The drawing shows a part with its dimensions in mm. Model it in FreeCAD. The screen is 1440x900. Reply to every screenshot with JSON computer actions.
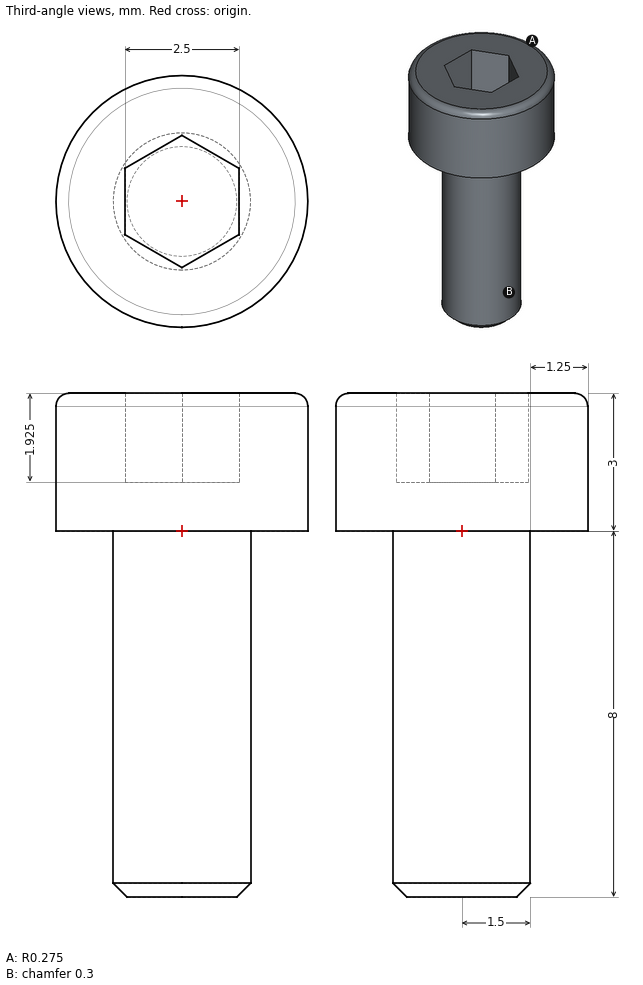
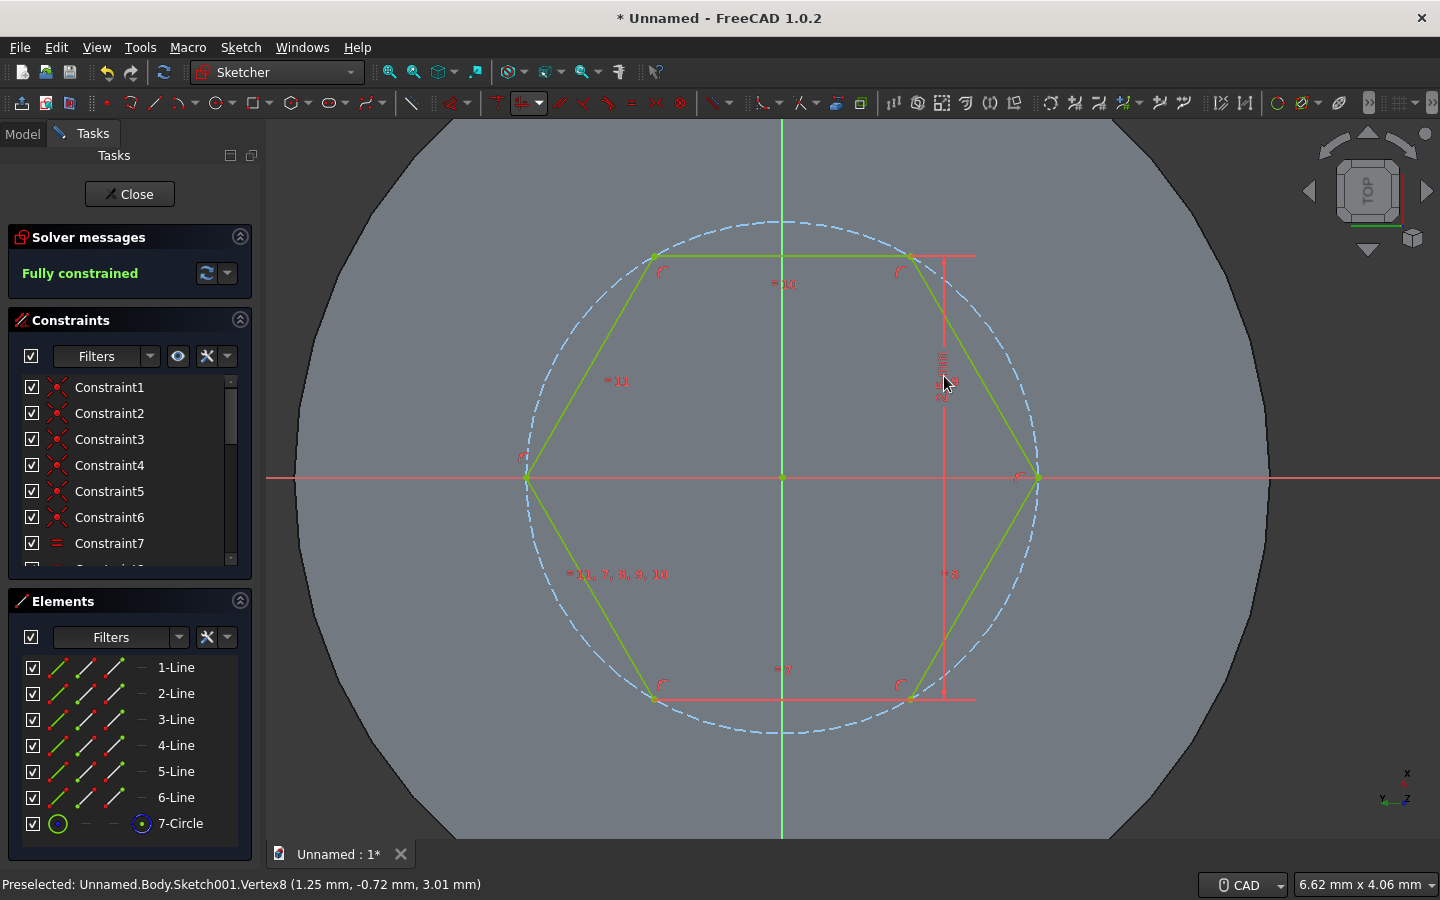
{"action": "left_click", "coordinate": [130, 194]}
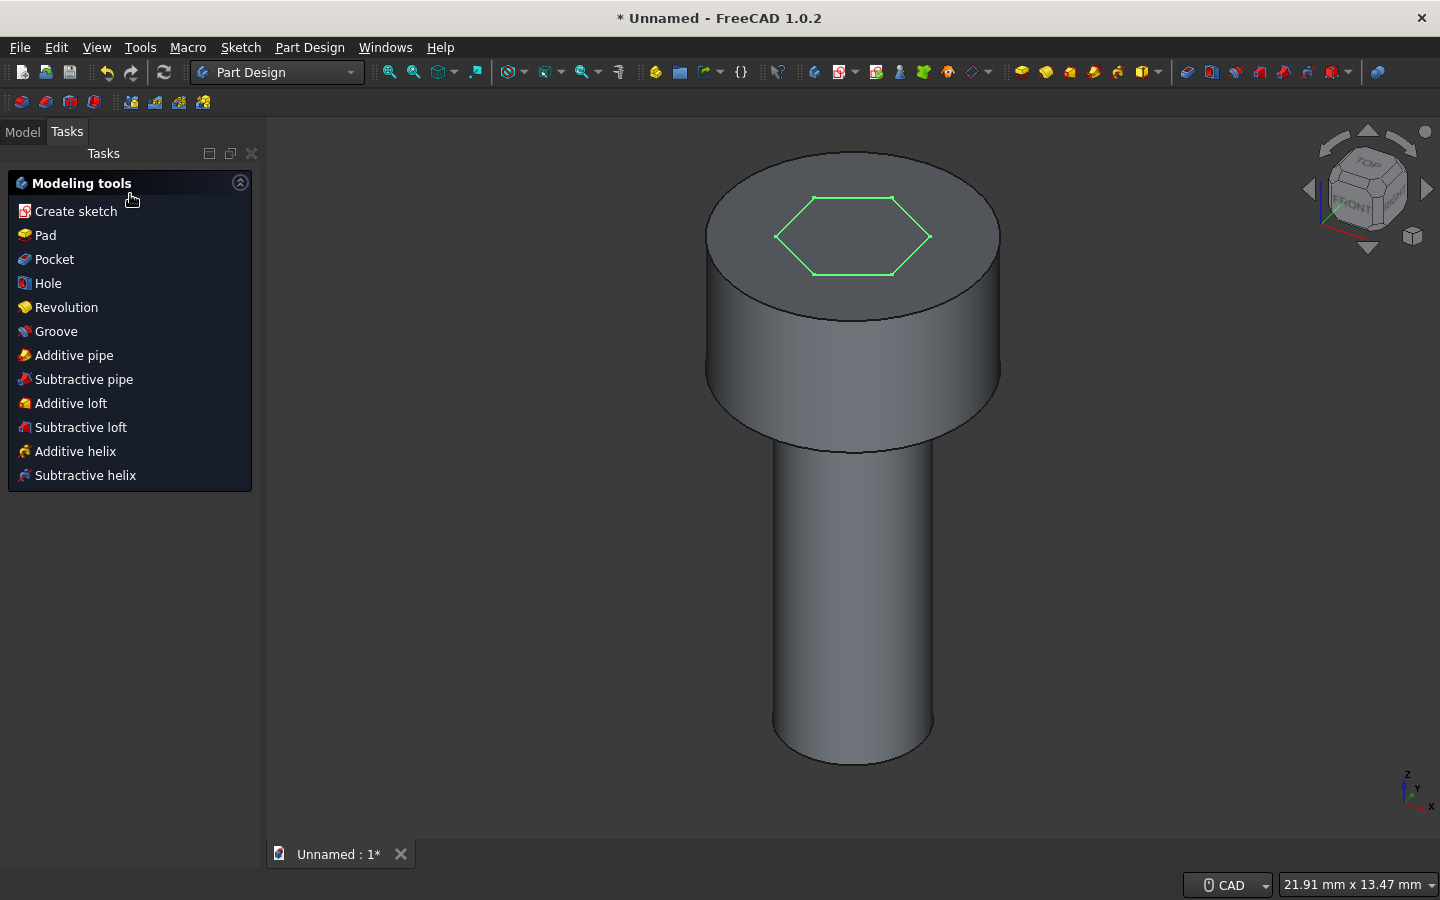
{"action": "left_click", "coordinate": [1188, 72]}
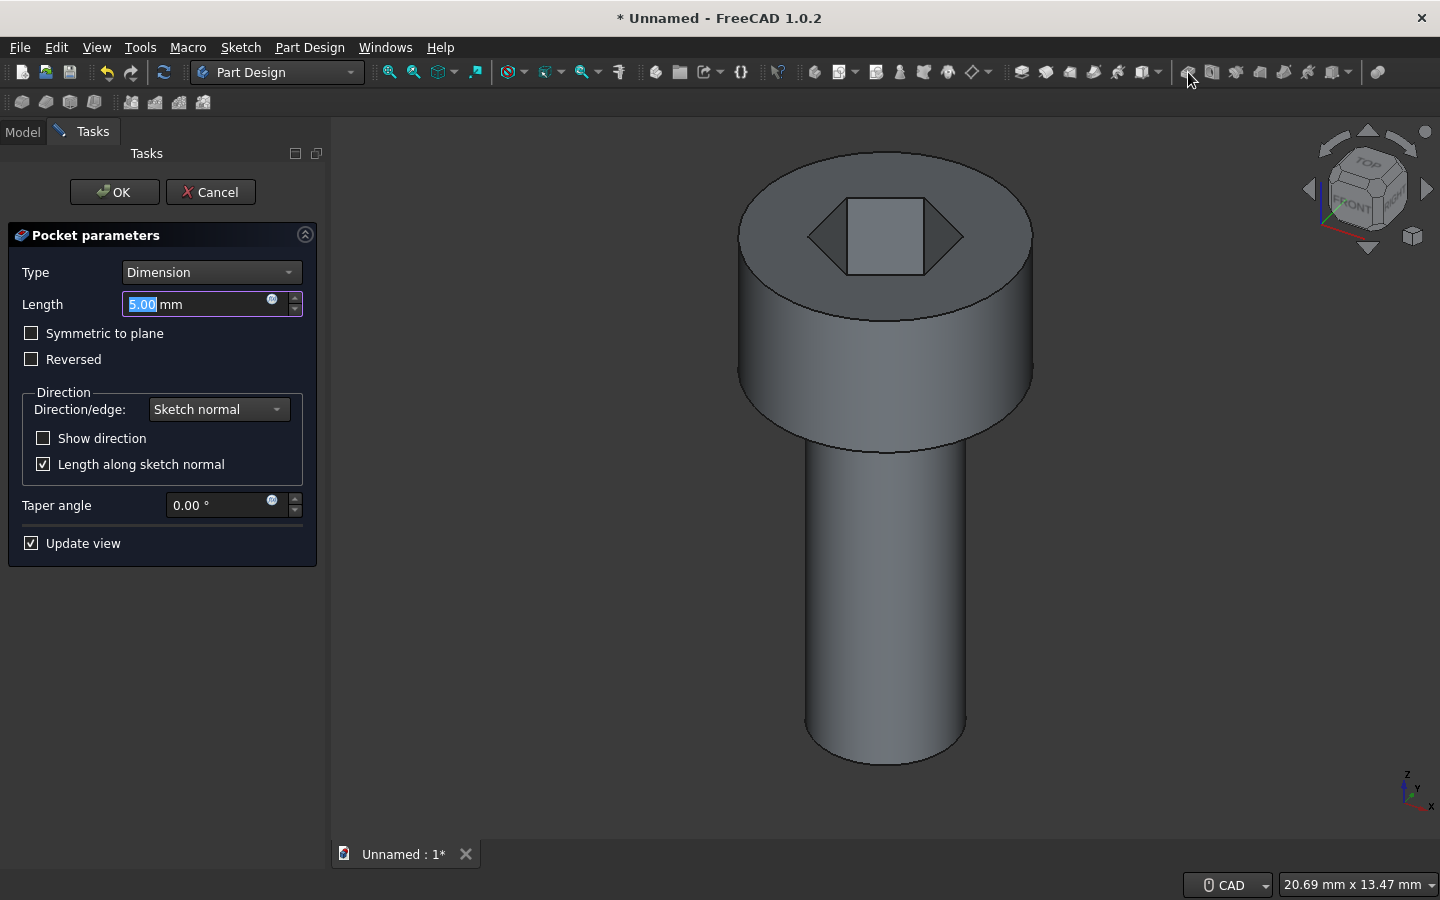
{"action": "type", "text": "1.925"}
{"action": "key", "text": "Tab"}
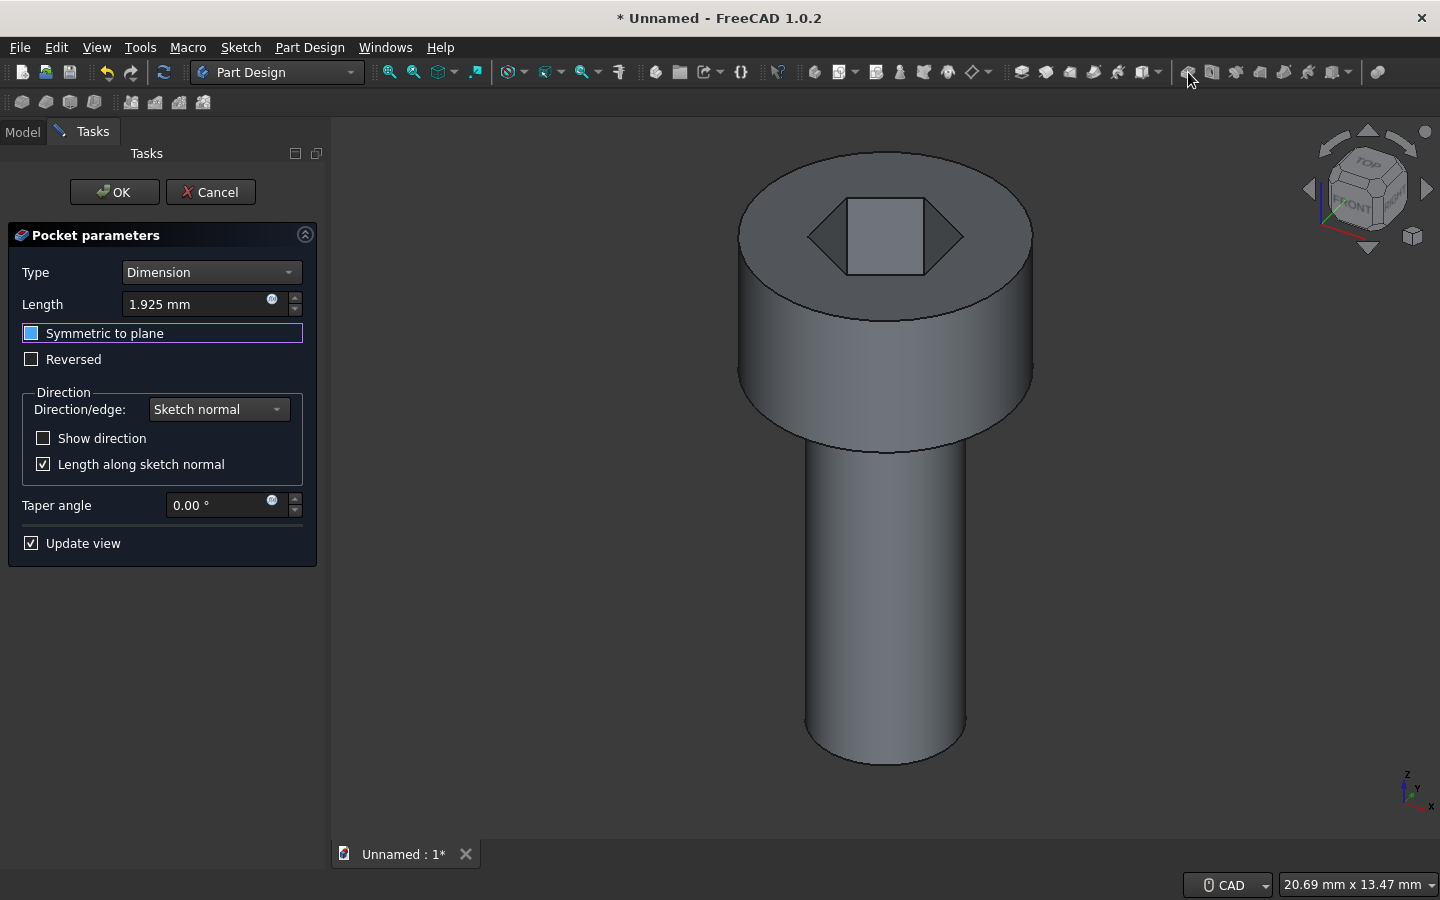
{"action": "left_click", "coordinate": [115, 192]}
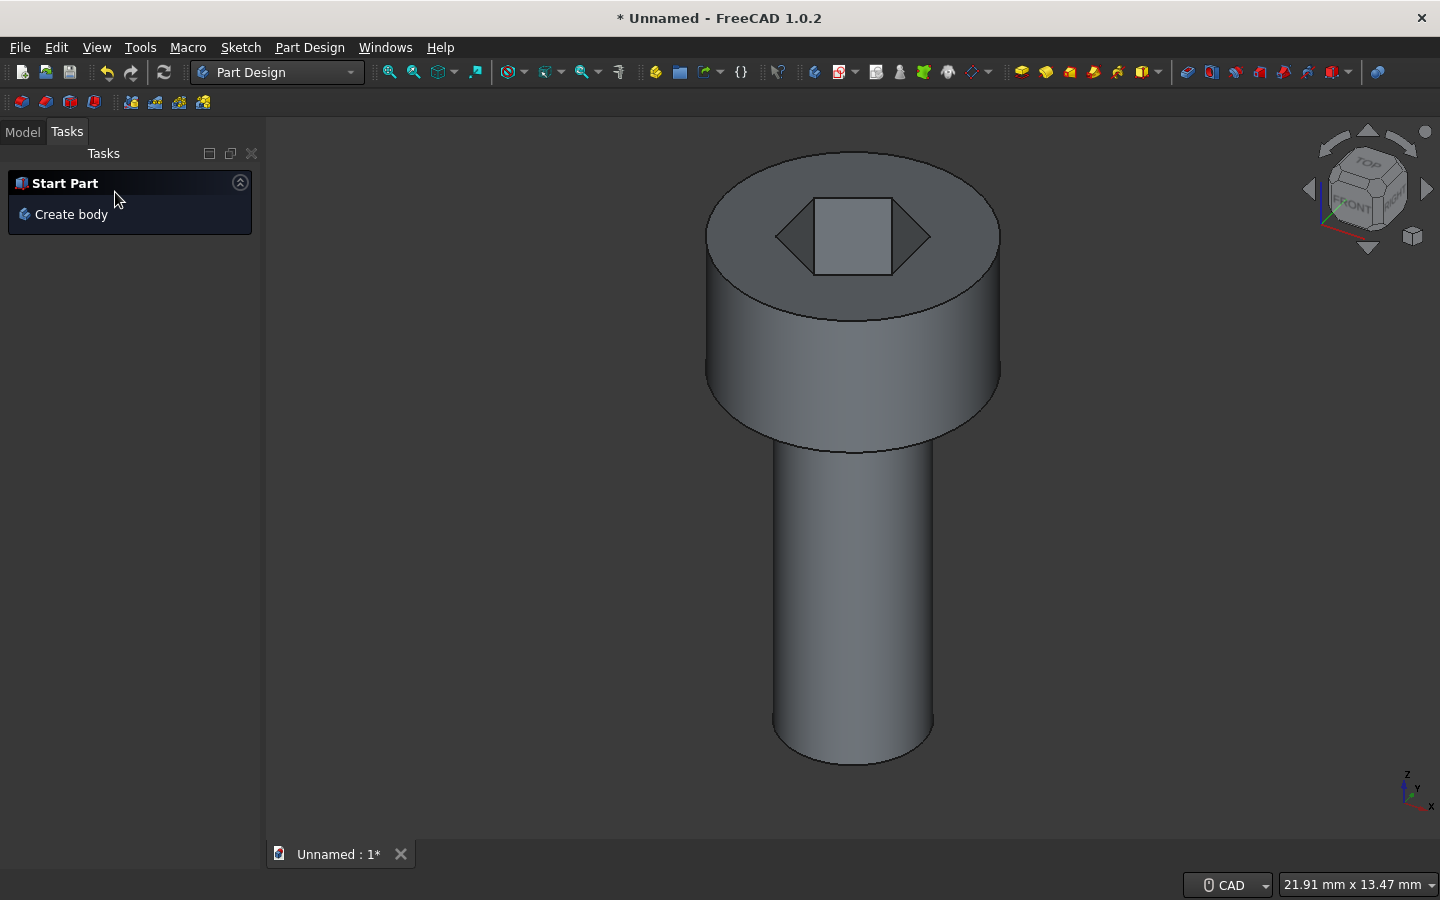
{"action": "left_click", "coordinate": [779, 309]}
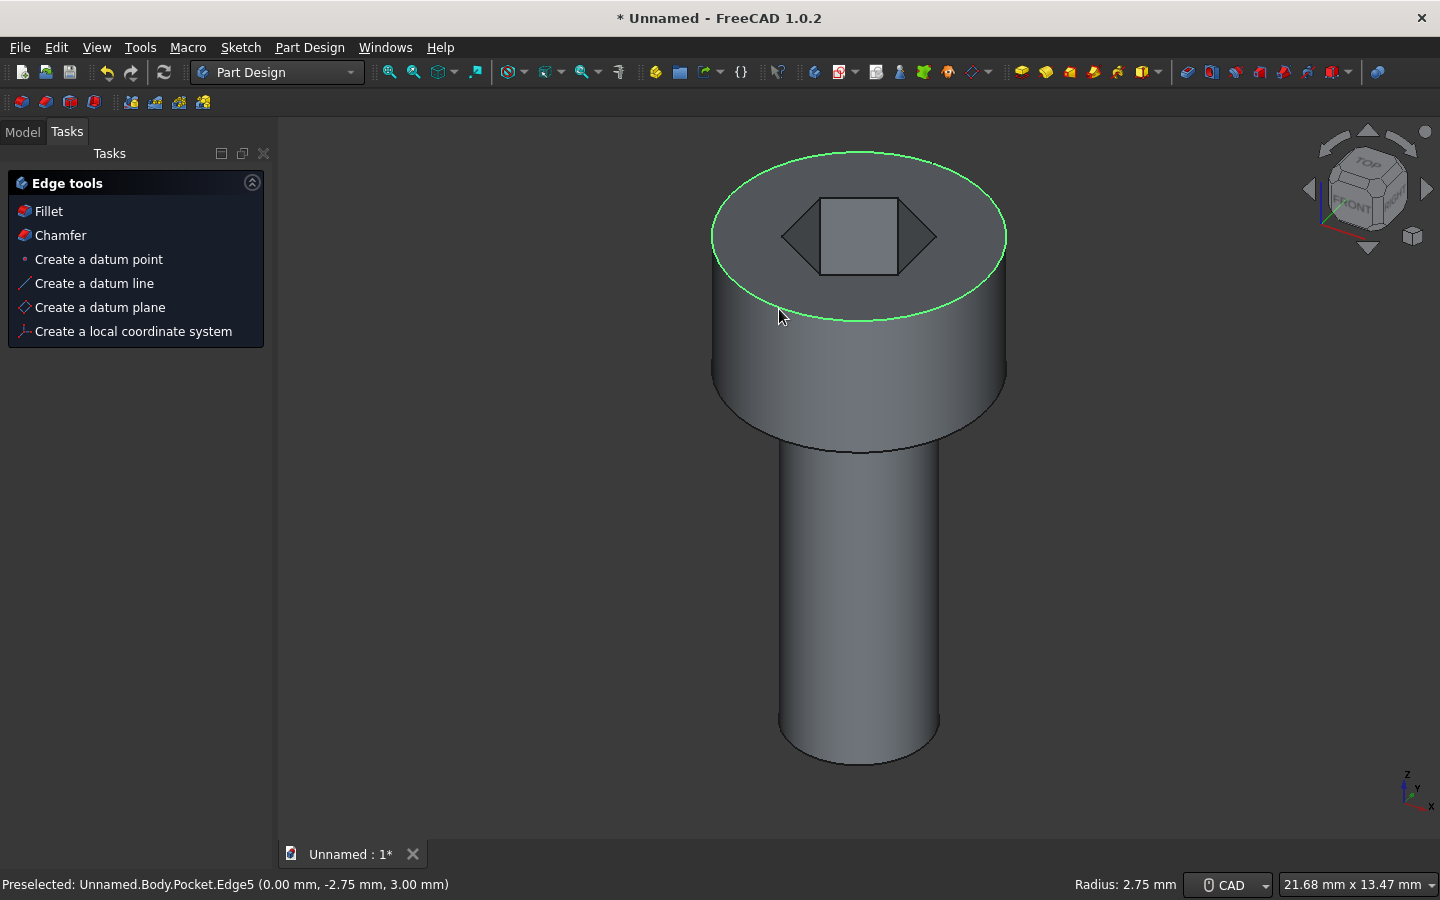
{"action": "left_click", "coordinate": [22, 102]}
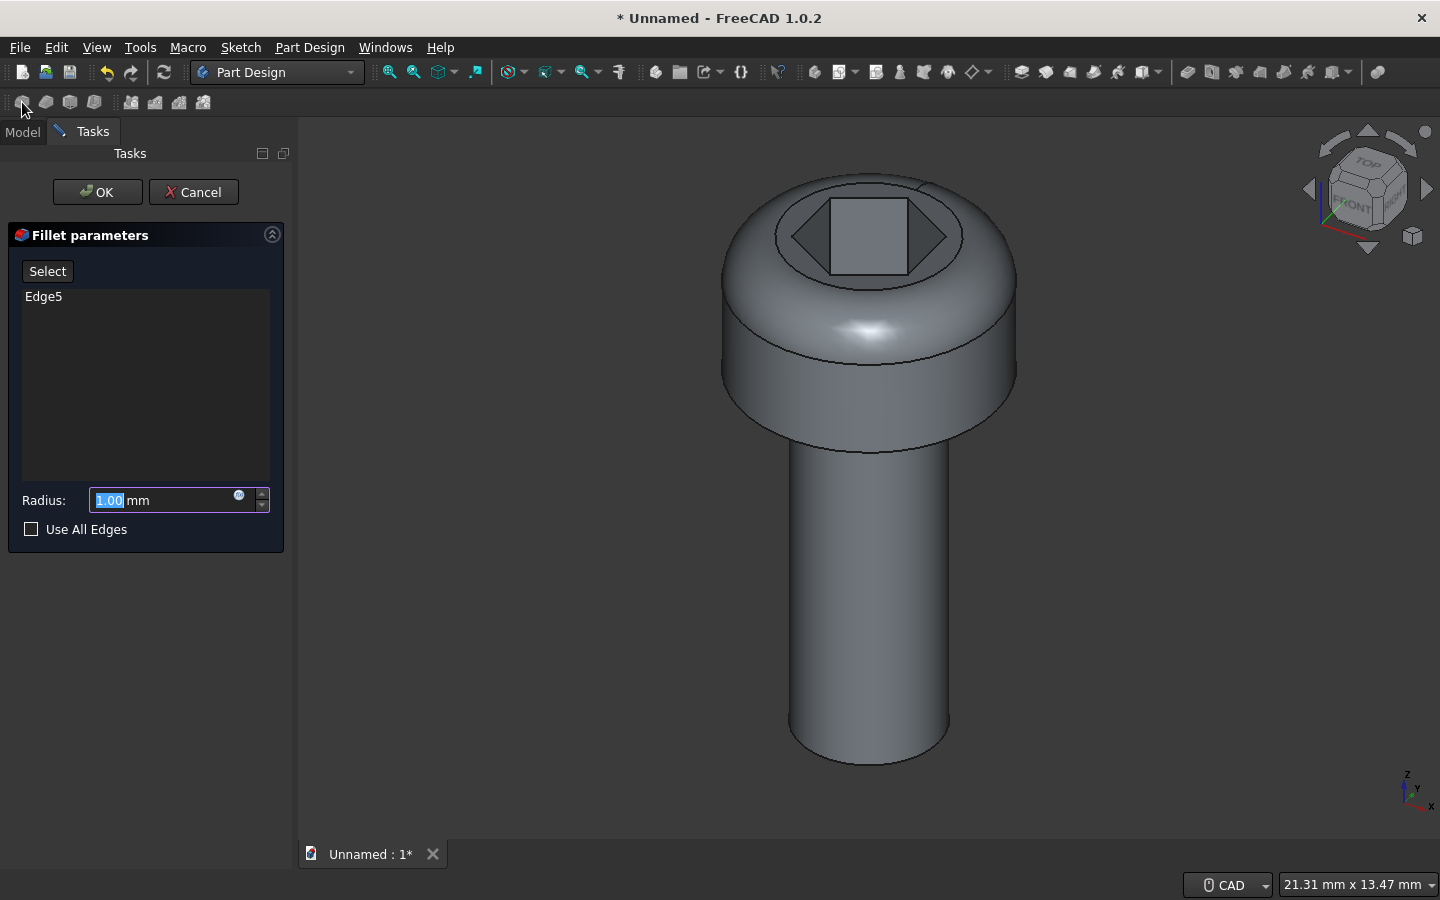
{"action": "type", "text": "0.275"}
{"action": "key", "text": "Tab"}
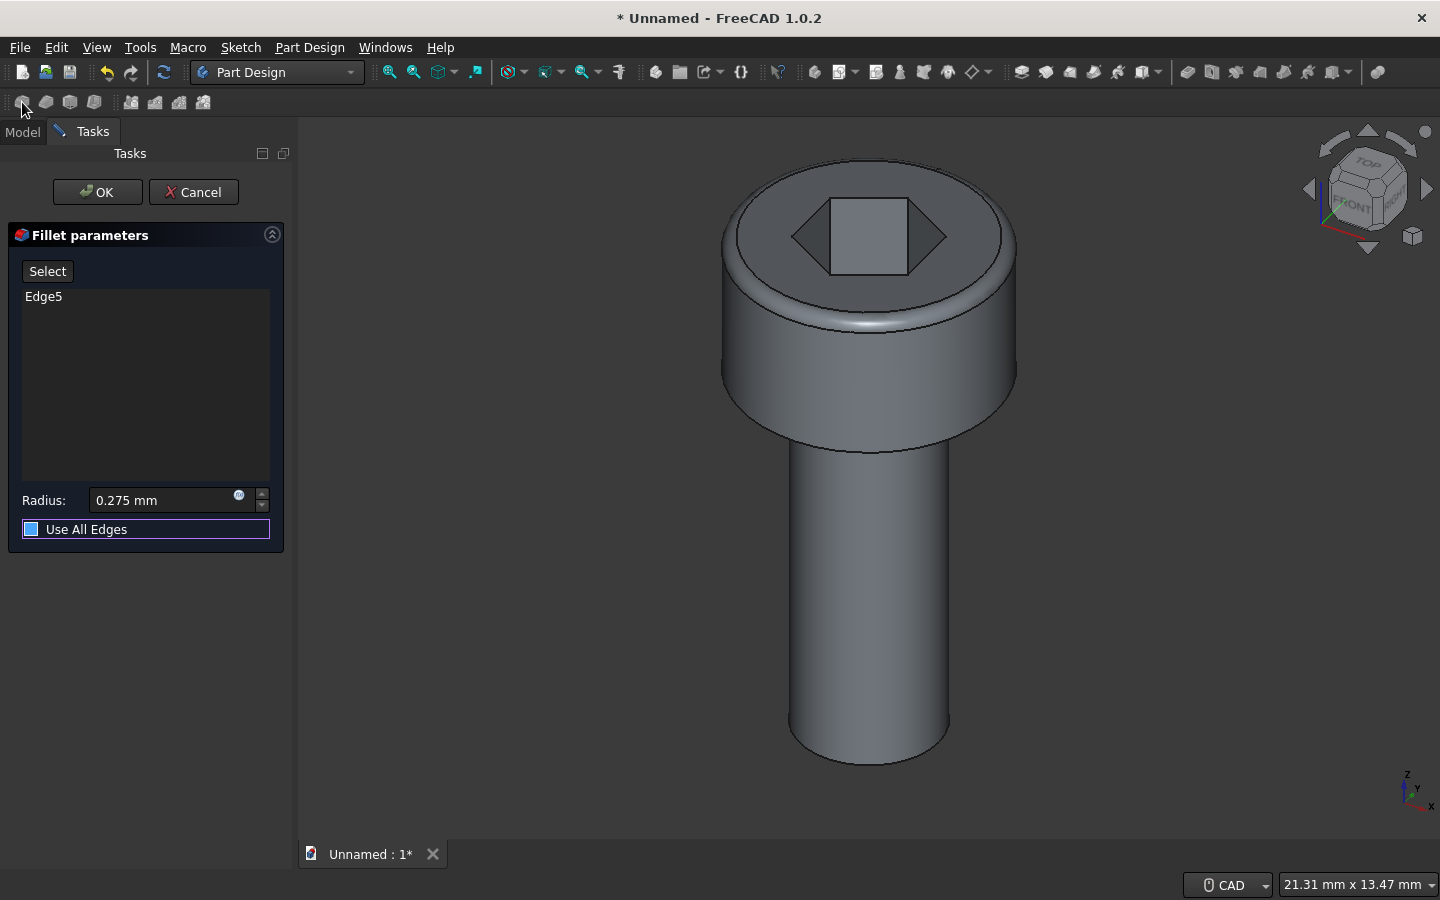
{"action": "left_click", "coordinate": [98, 192]}